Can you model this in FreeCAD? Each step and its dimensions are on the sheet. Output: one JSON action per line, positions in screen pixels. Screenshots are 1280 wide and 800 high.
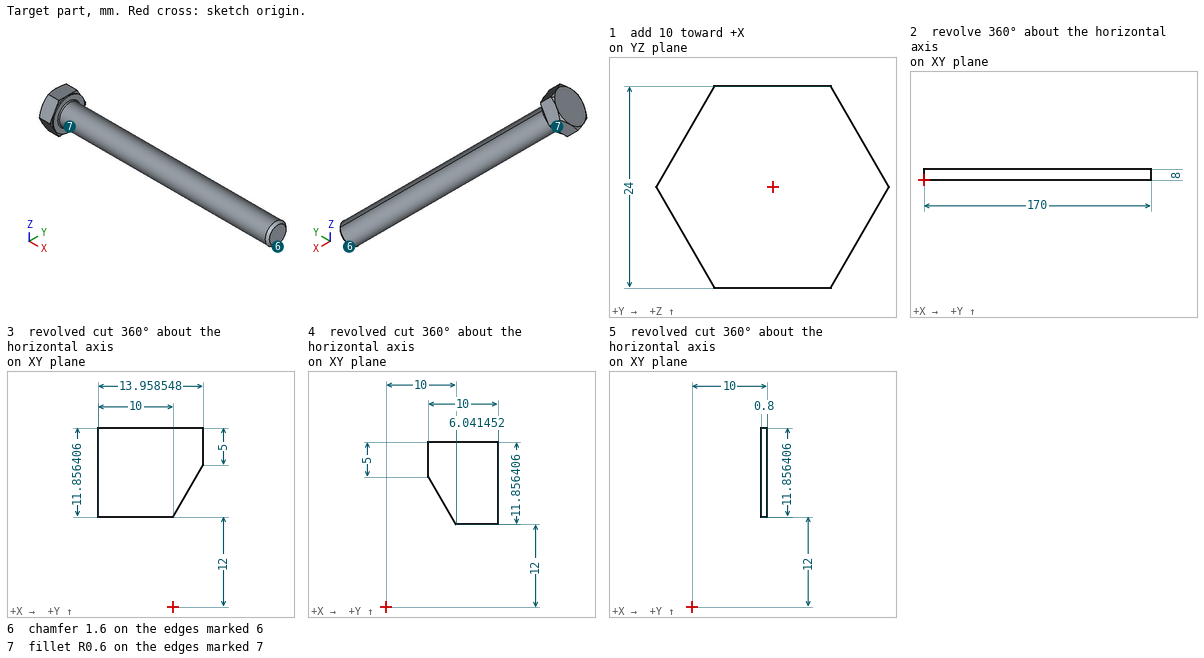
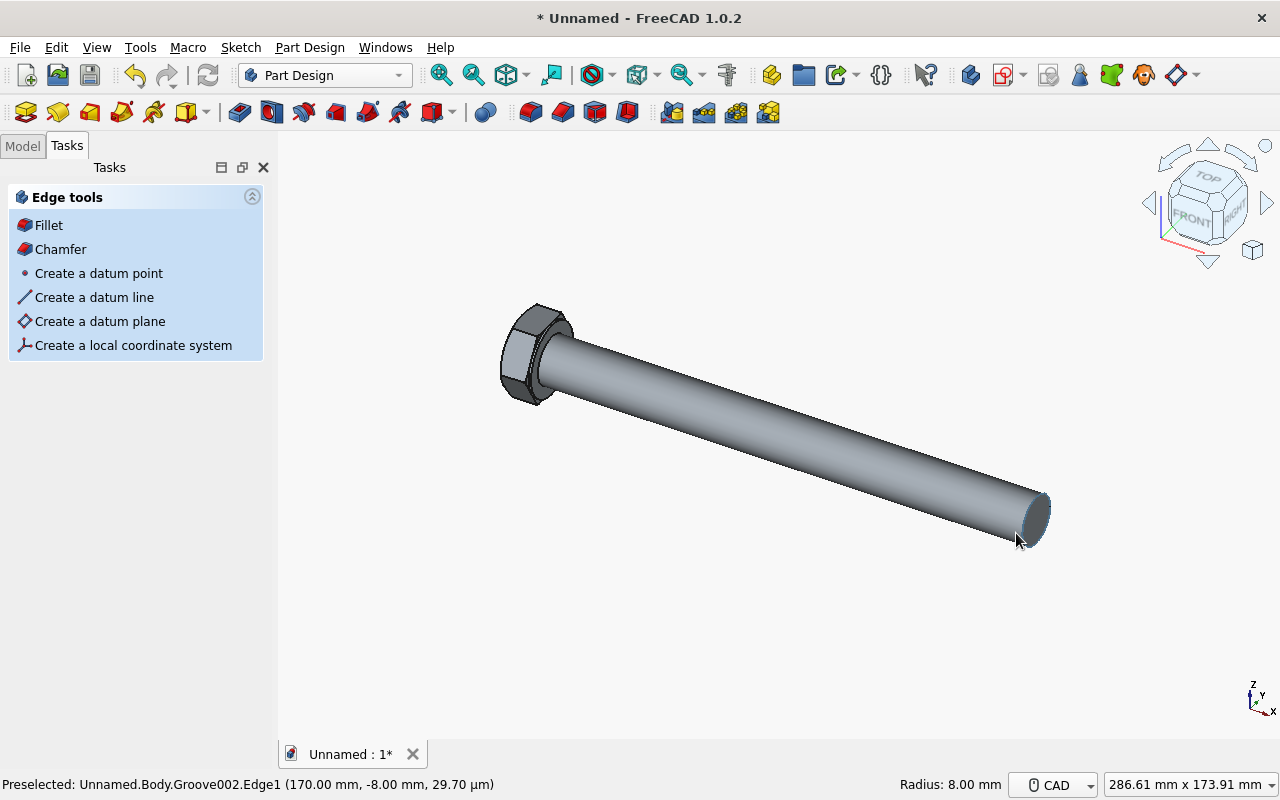
{"action": "left_click", "coordinate": [564, 112]}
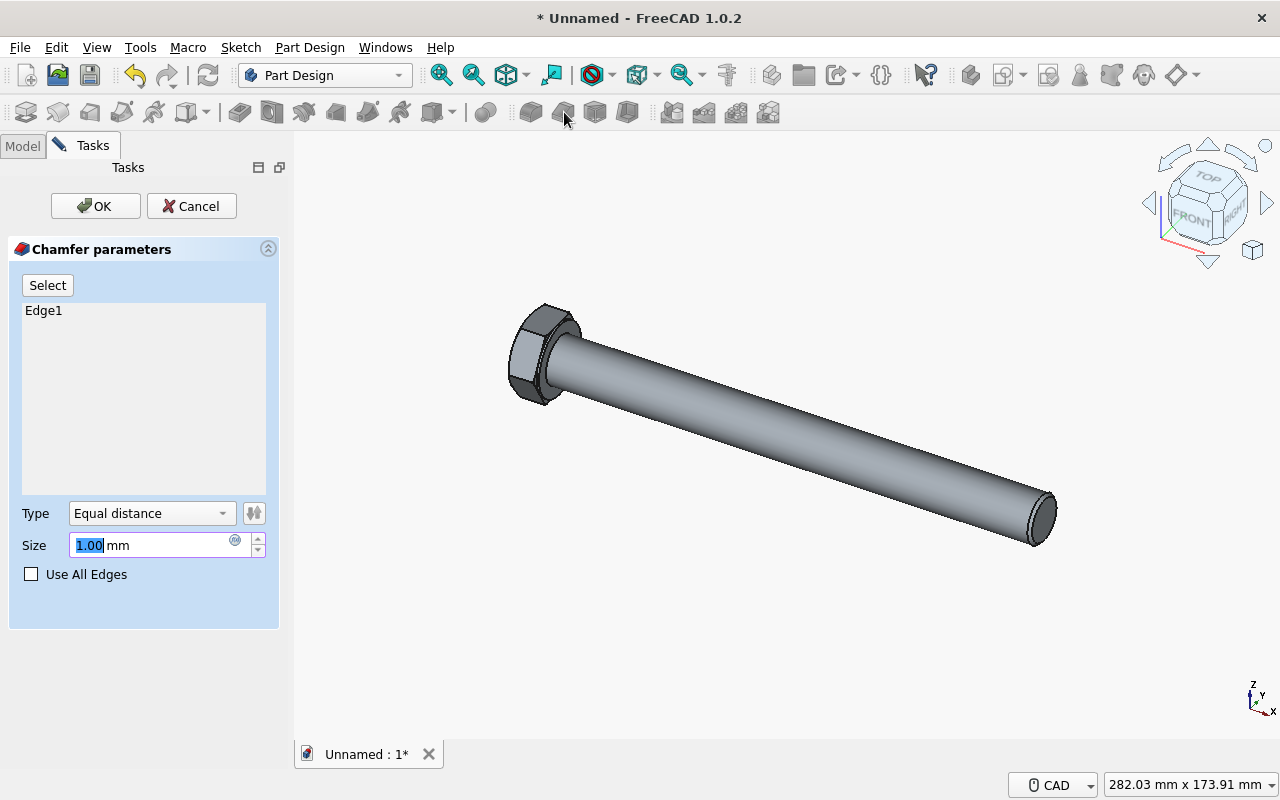
{"action": "type", "text": "1.6"}
{"action": "key", "text": "Tab"}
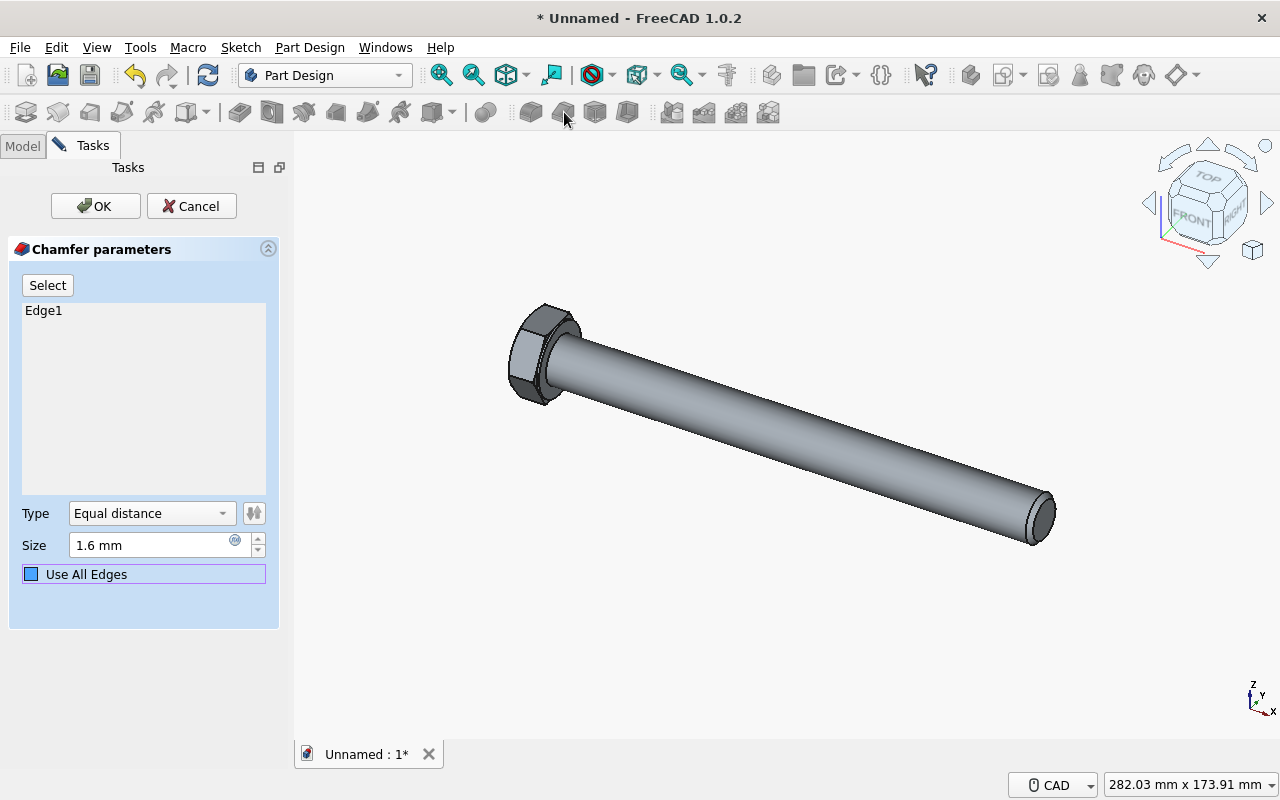
{"action": "left_click", "coordinate": [96, 206]}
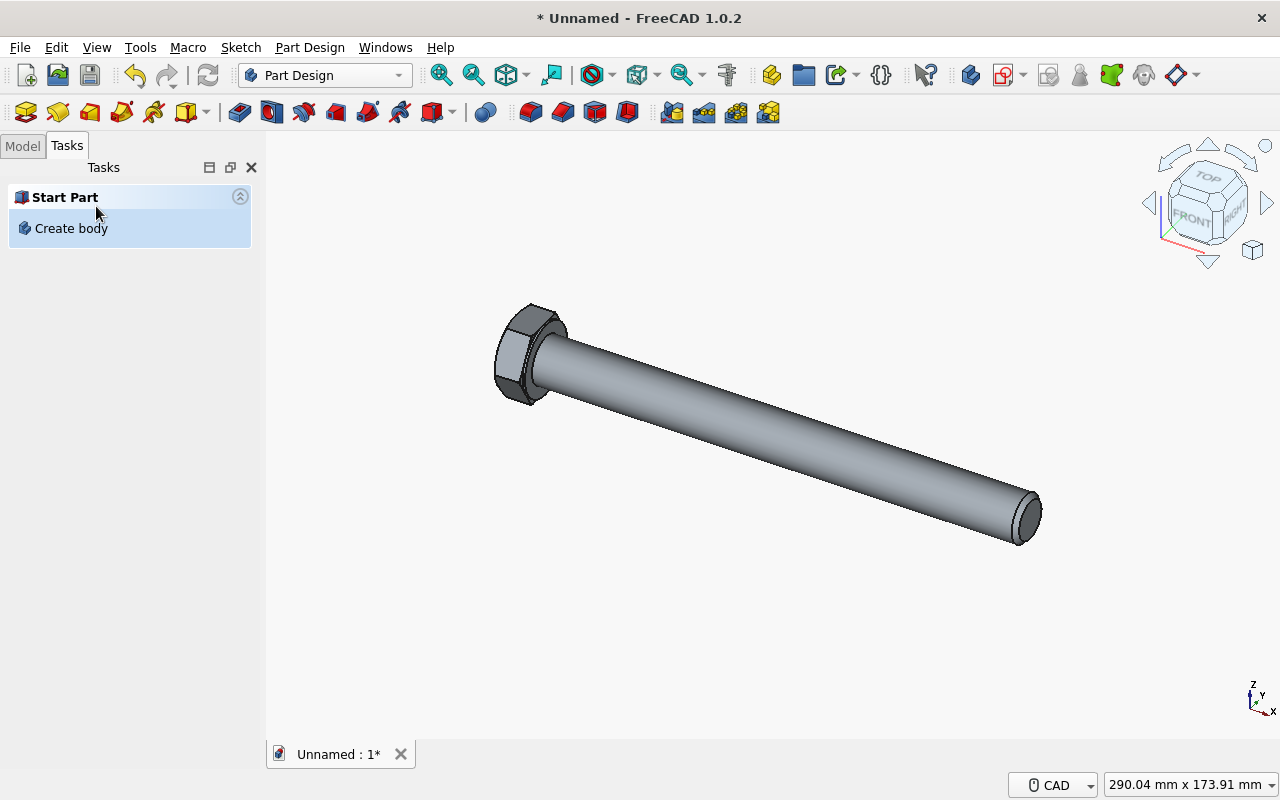
{"action": "key", "text": "0"}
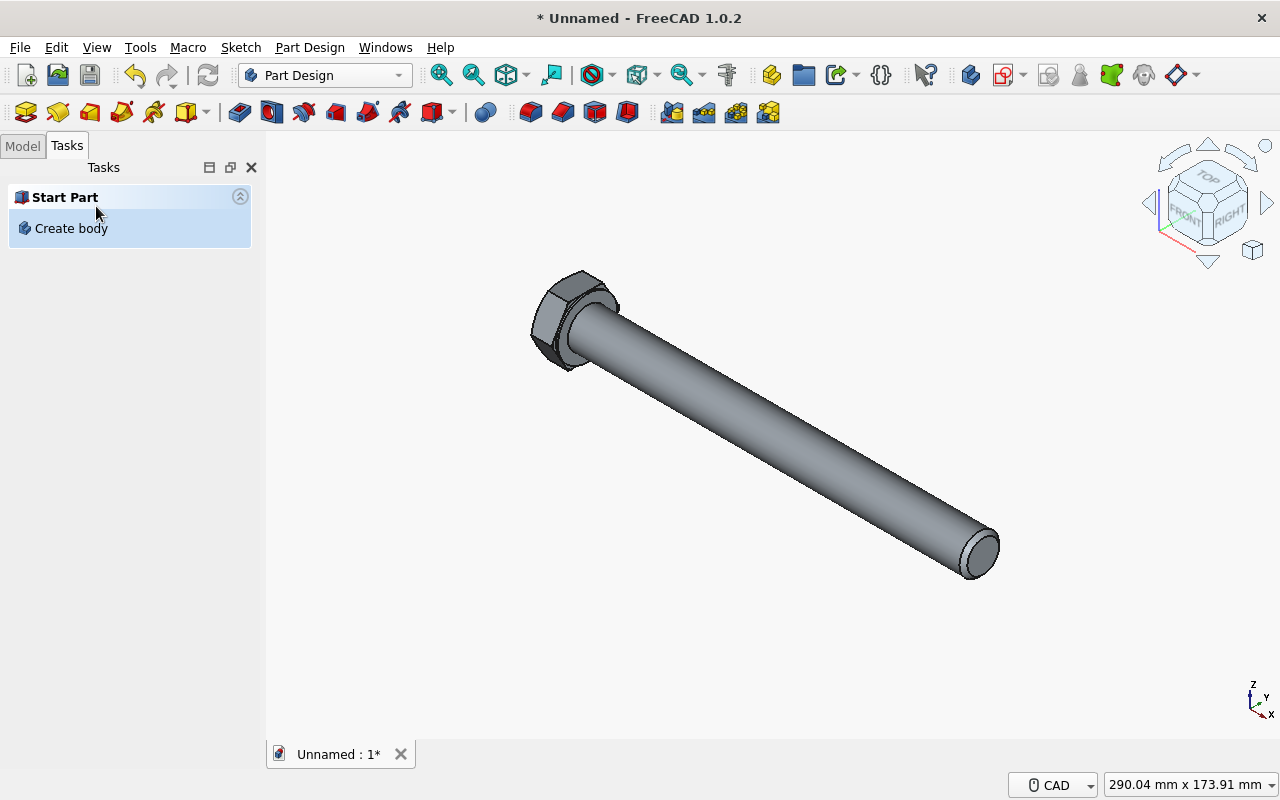
{"action": "key", "text": "2"}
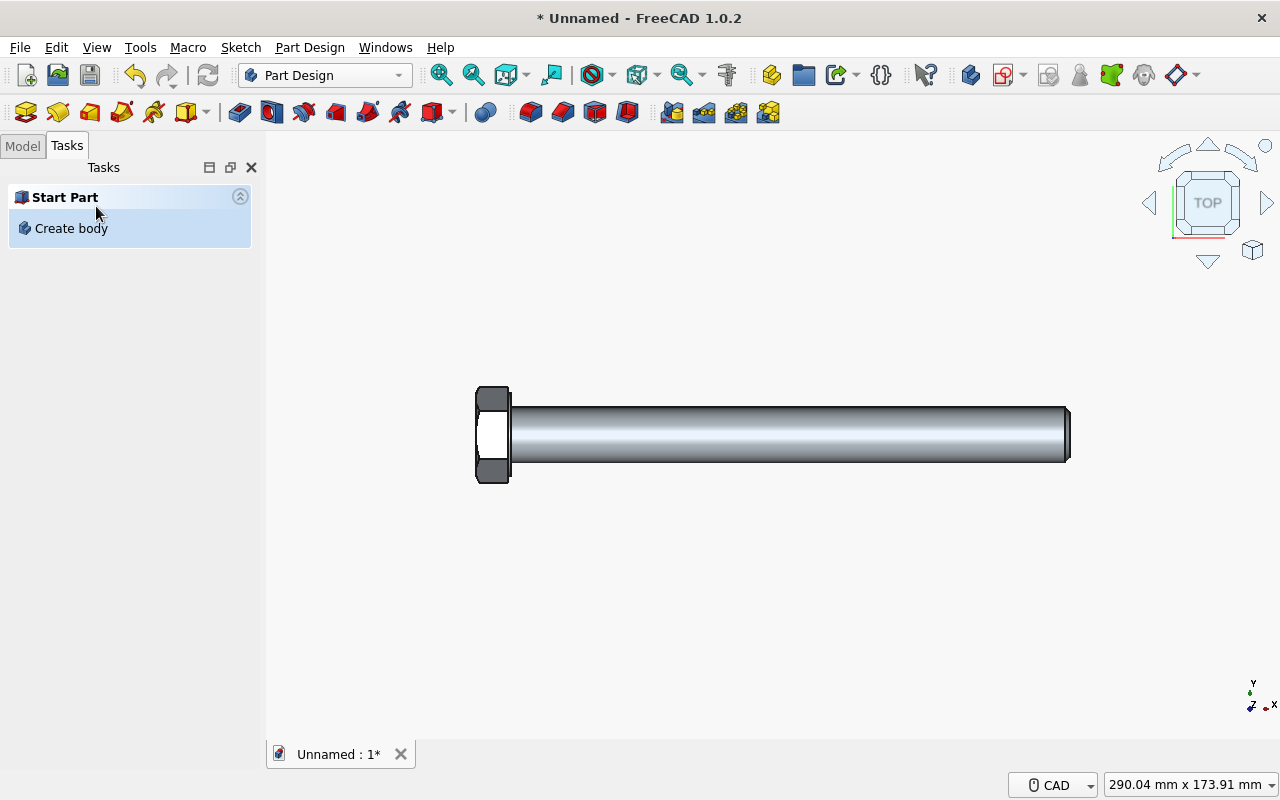
{"action": "key", "text": "1"}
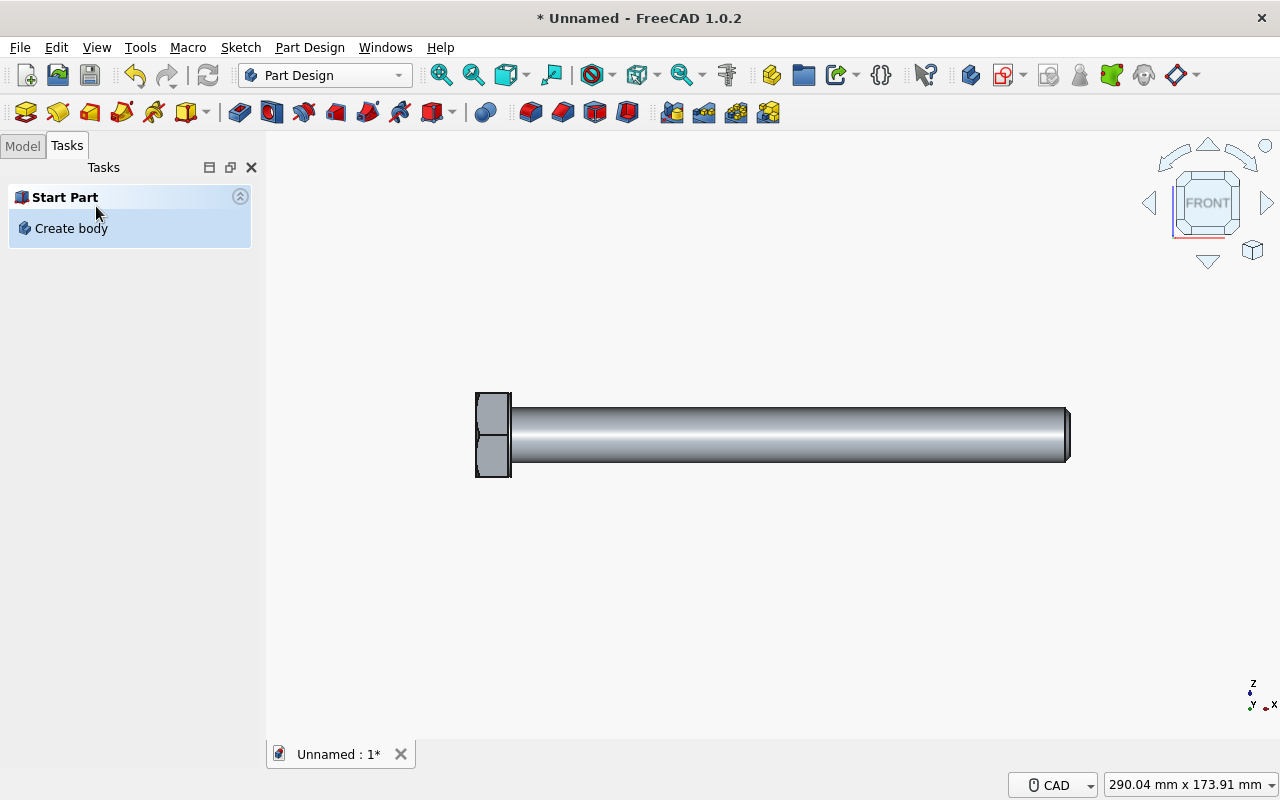
{"action": "key", "text": "3"}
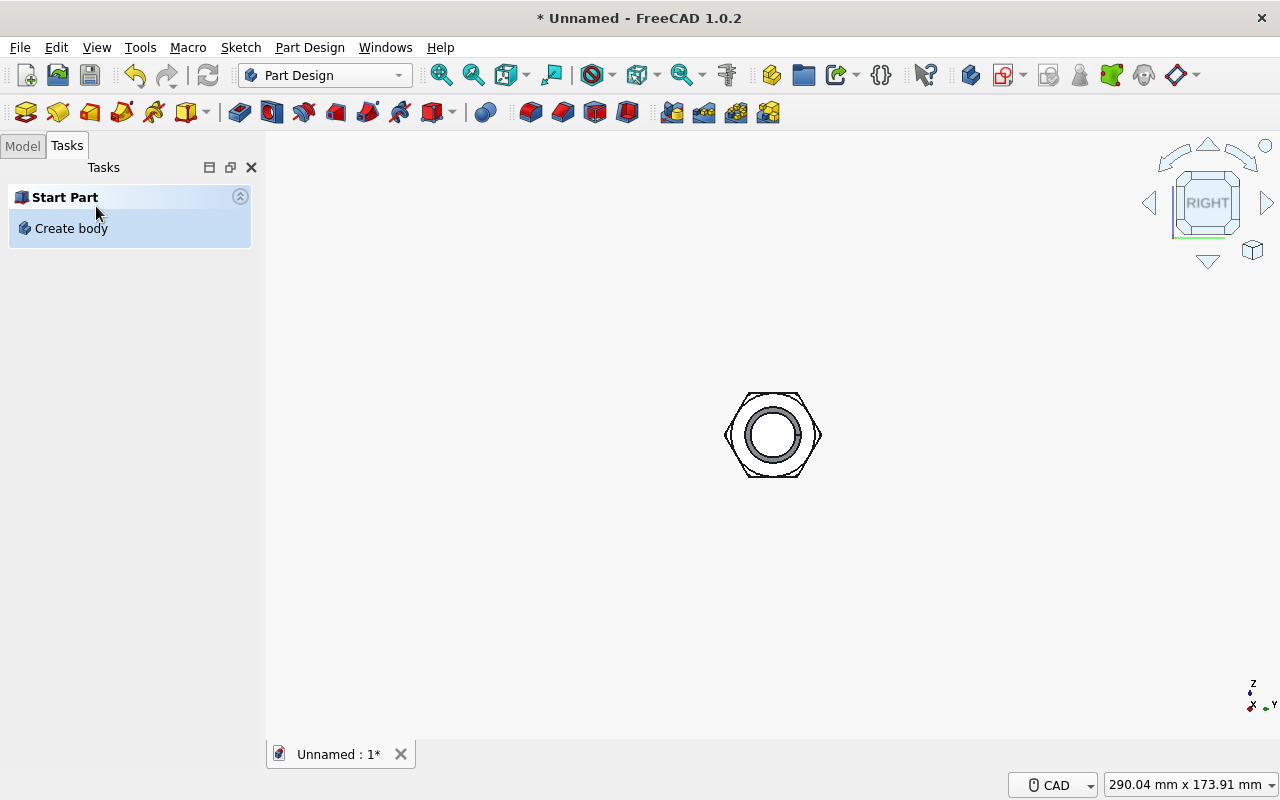
{"action": "left_click", "coordinate": [442, 76]}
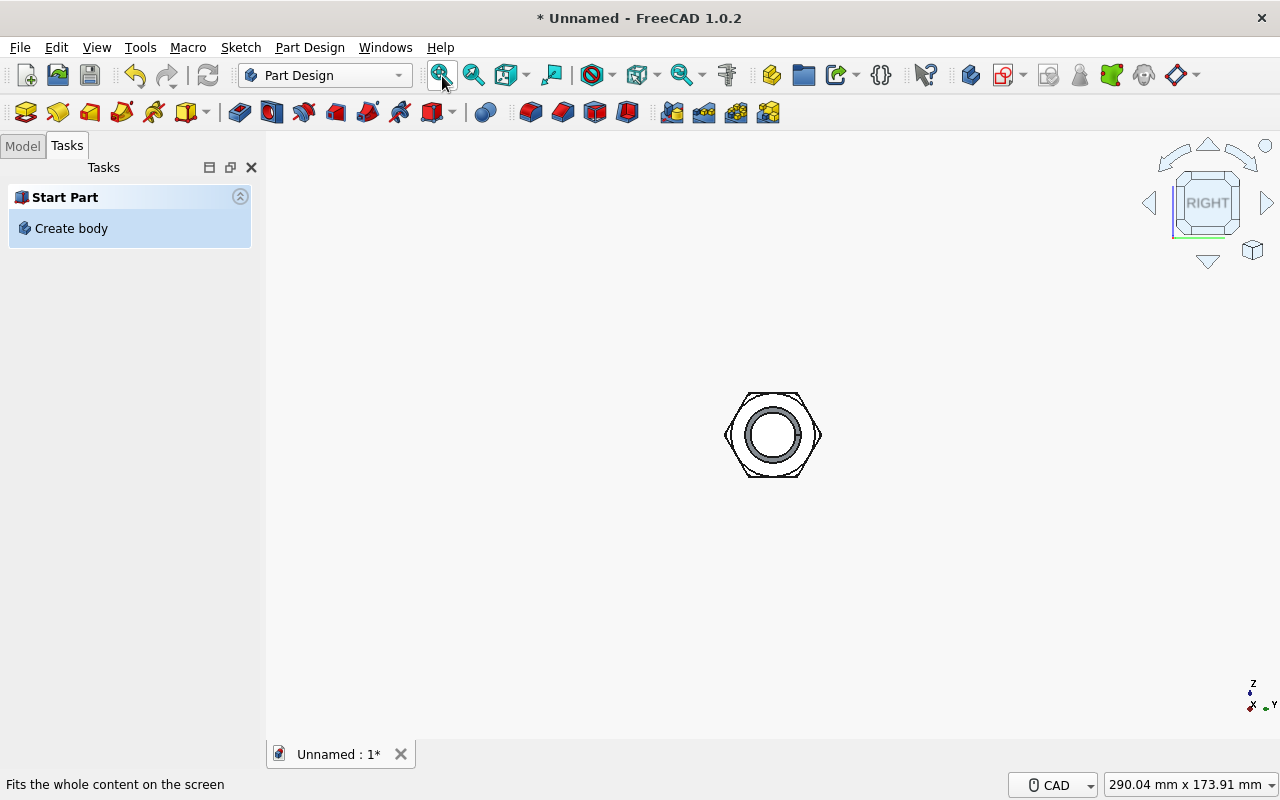
{"action": "key", "text": "5"}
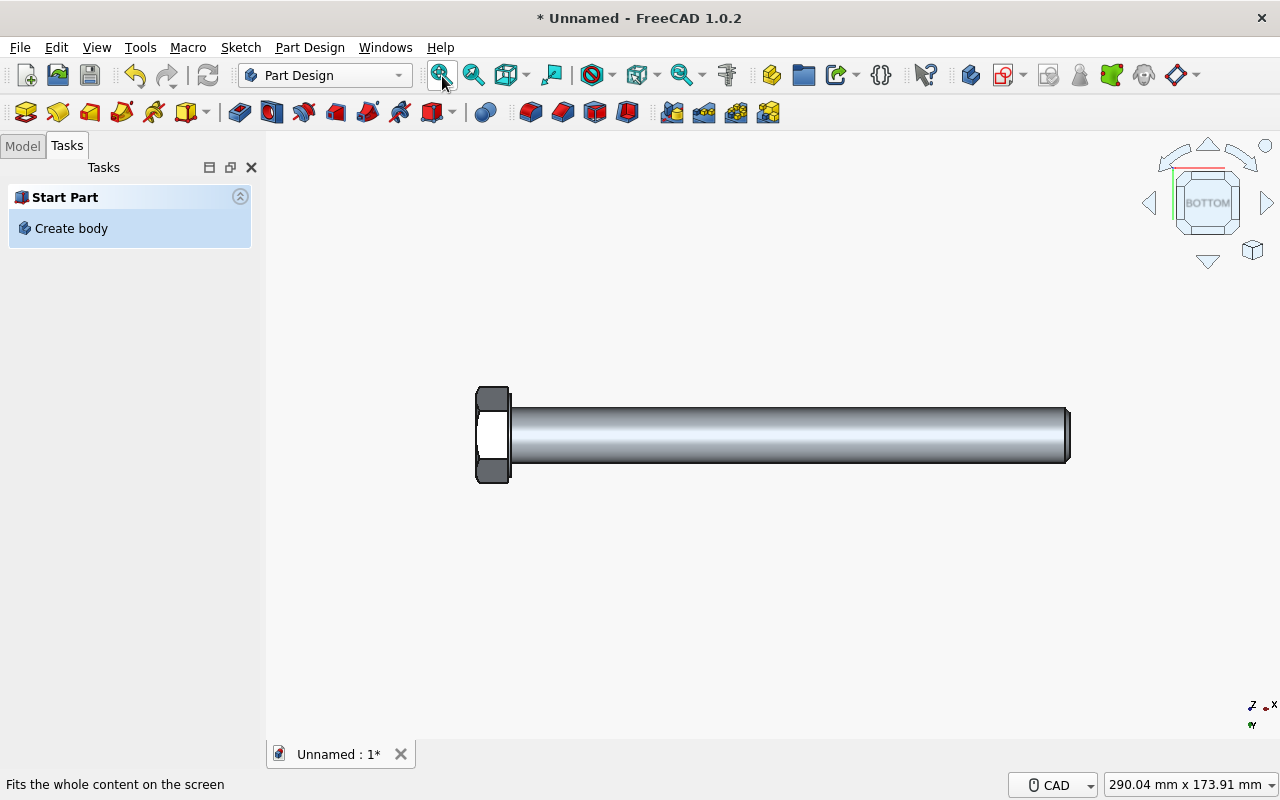
{"action": "key", "text": "4"}